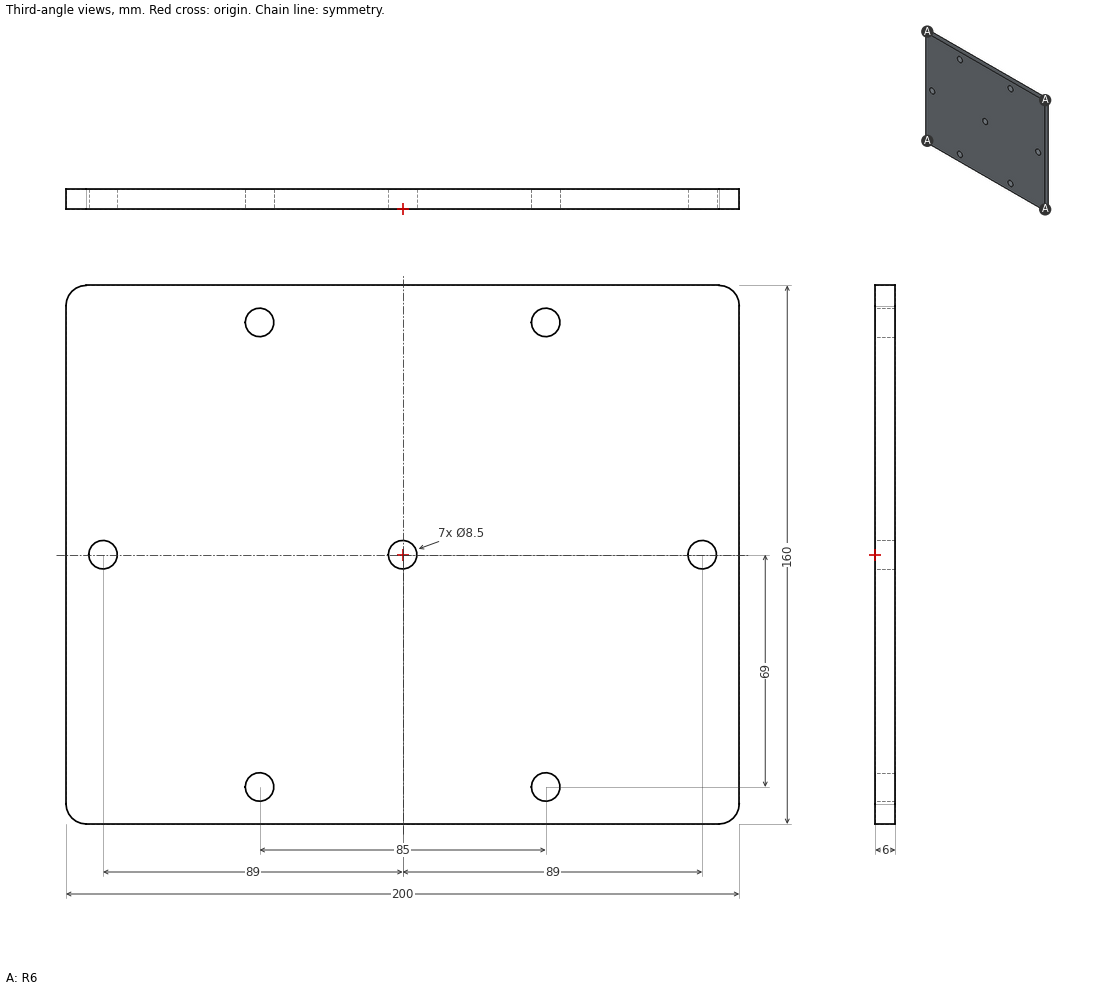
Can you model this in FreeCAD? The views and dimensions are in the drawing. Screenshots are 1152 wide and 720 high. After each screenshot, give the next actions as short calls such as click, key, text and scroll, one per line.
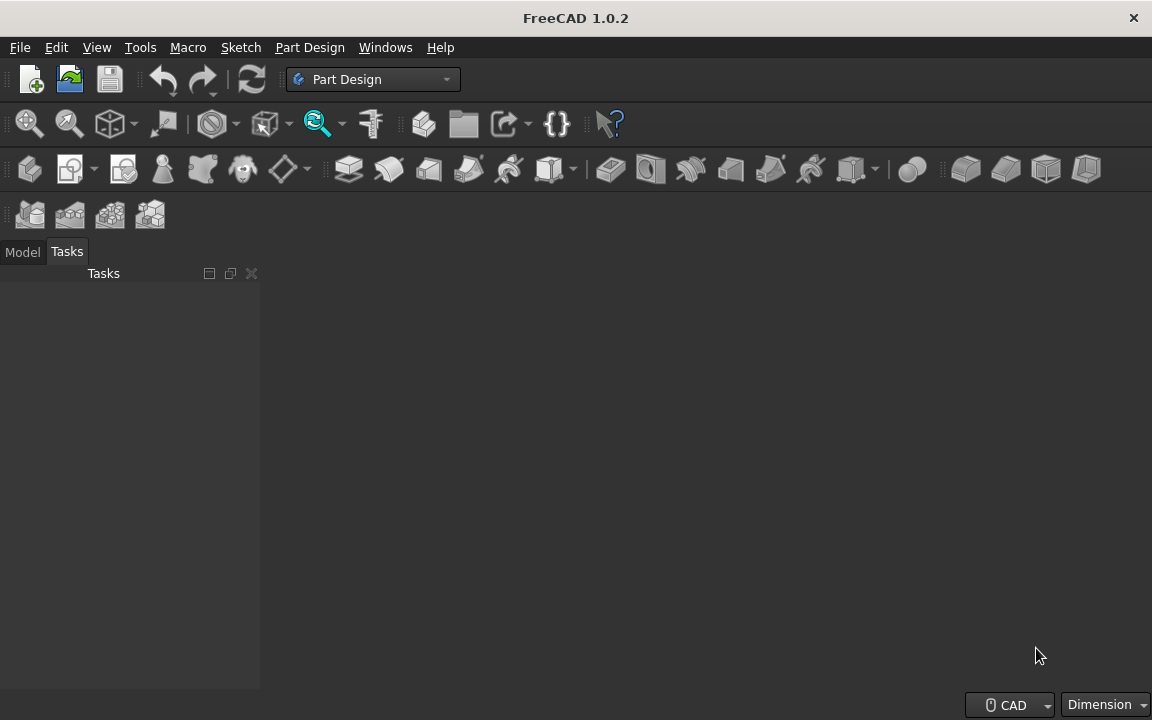
click(30, 80)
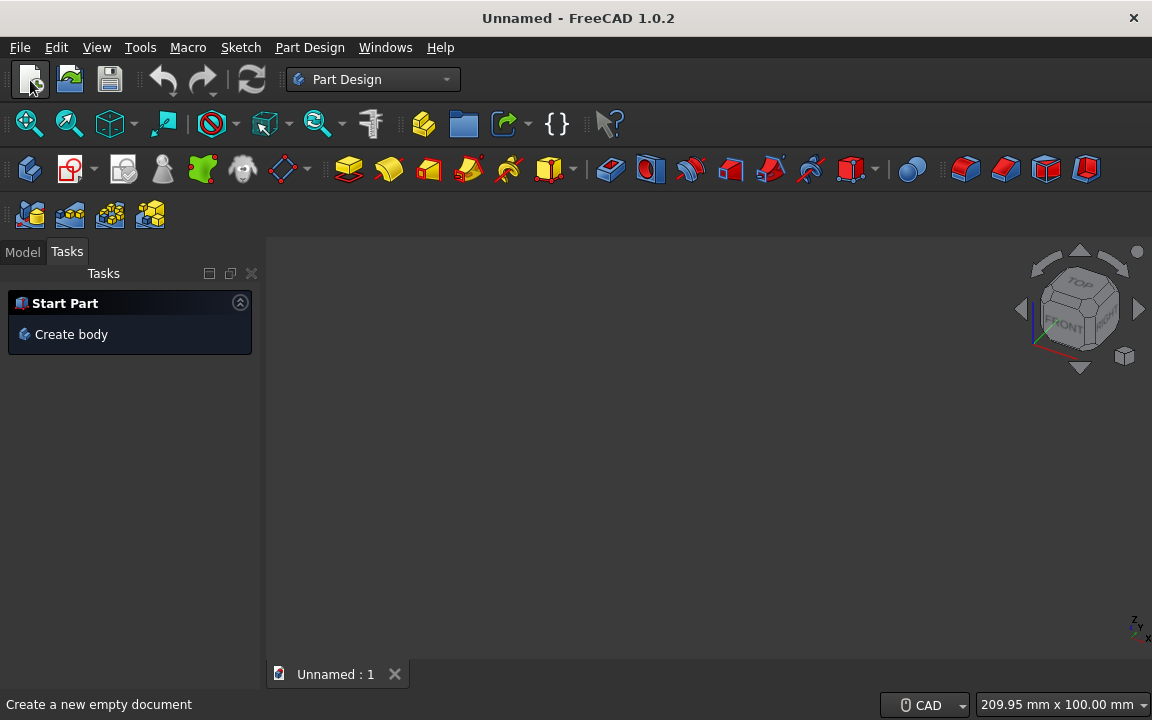
click(70, 170)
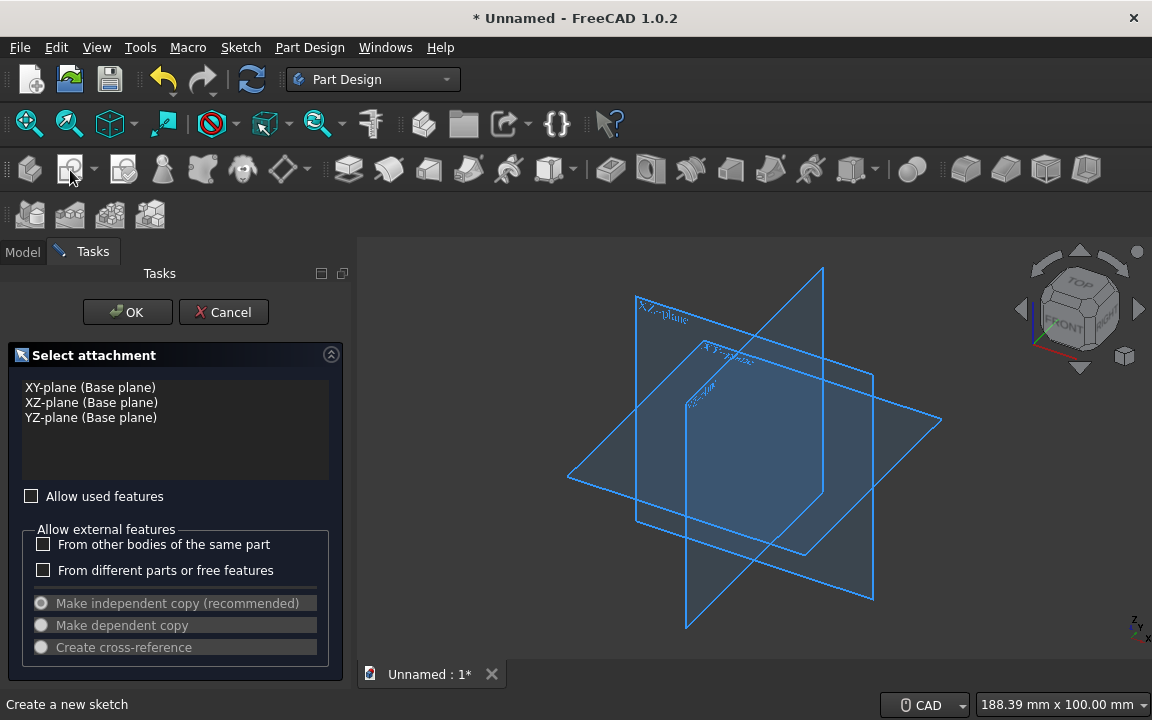
click(82, 402)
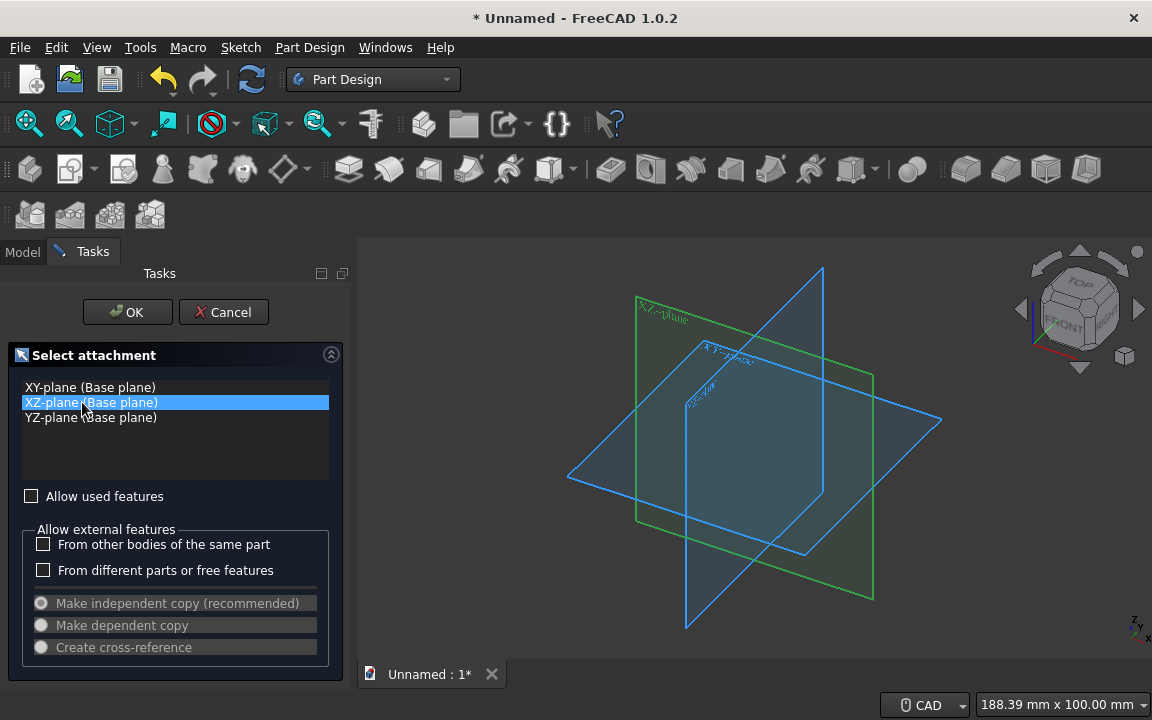
click(128, 312)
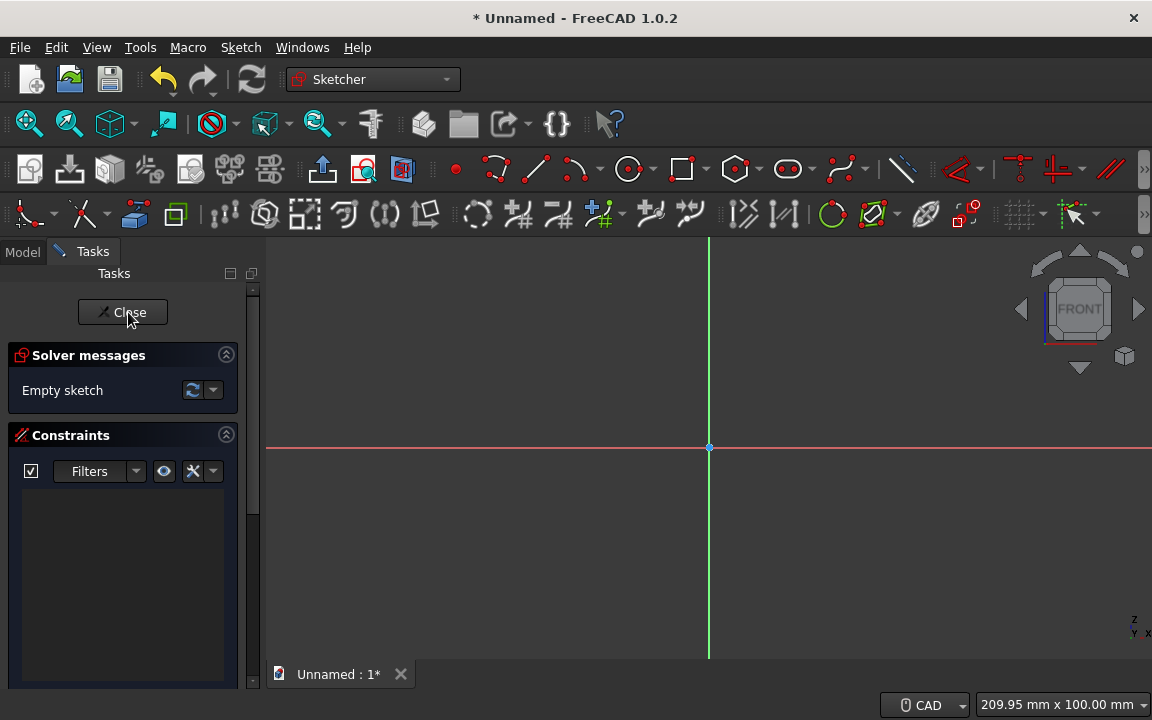
scroll(601, 448, down, 5)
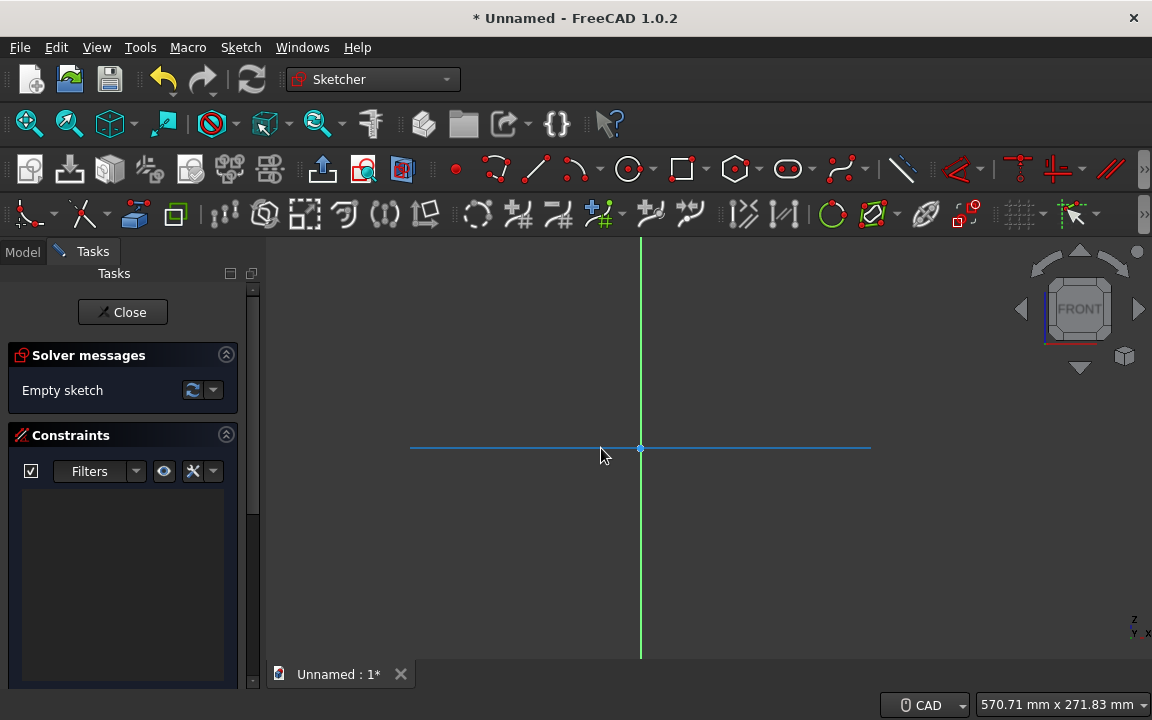
click(708, 170)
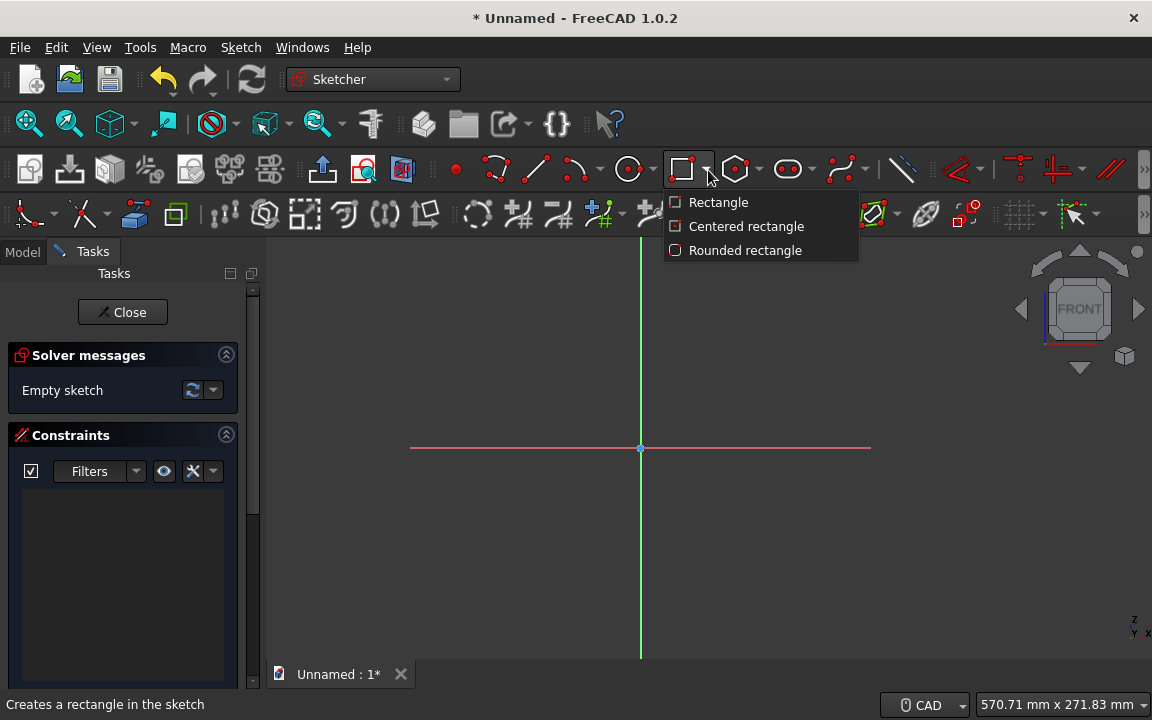
click(762, 226)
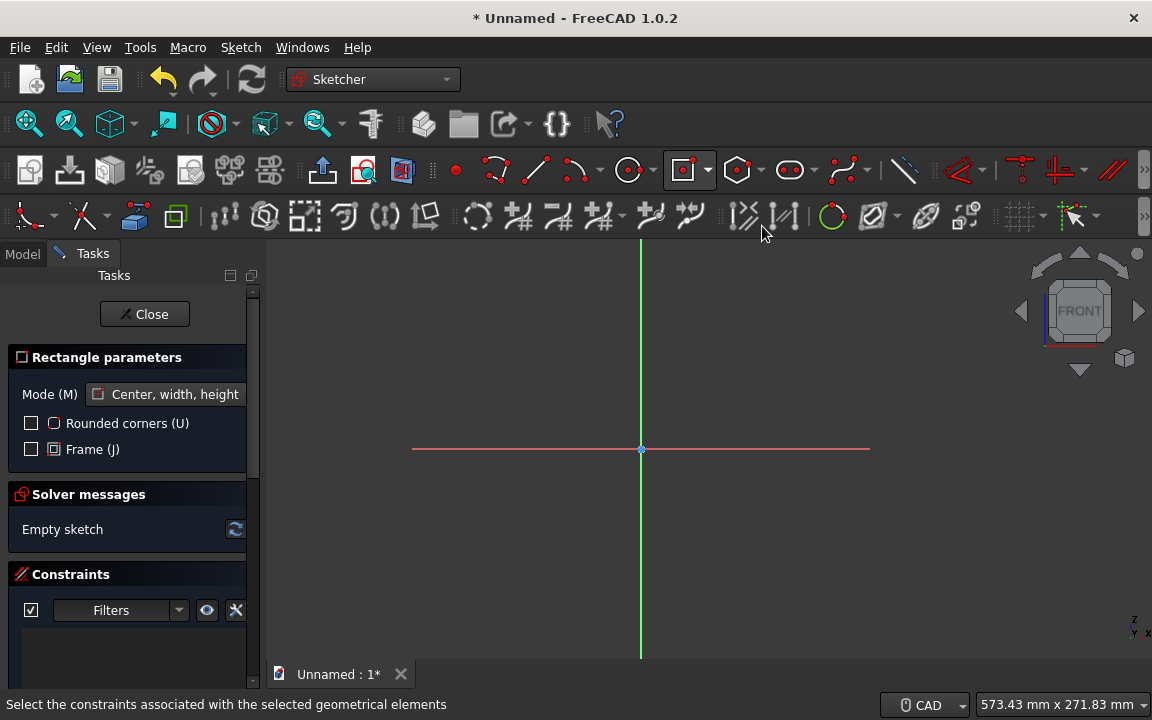
click(641, 449)
click(796, 326)
key(Escape)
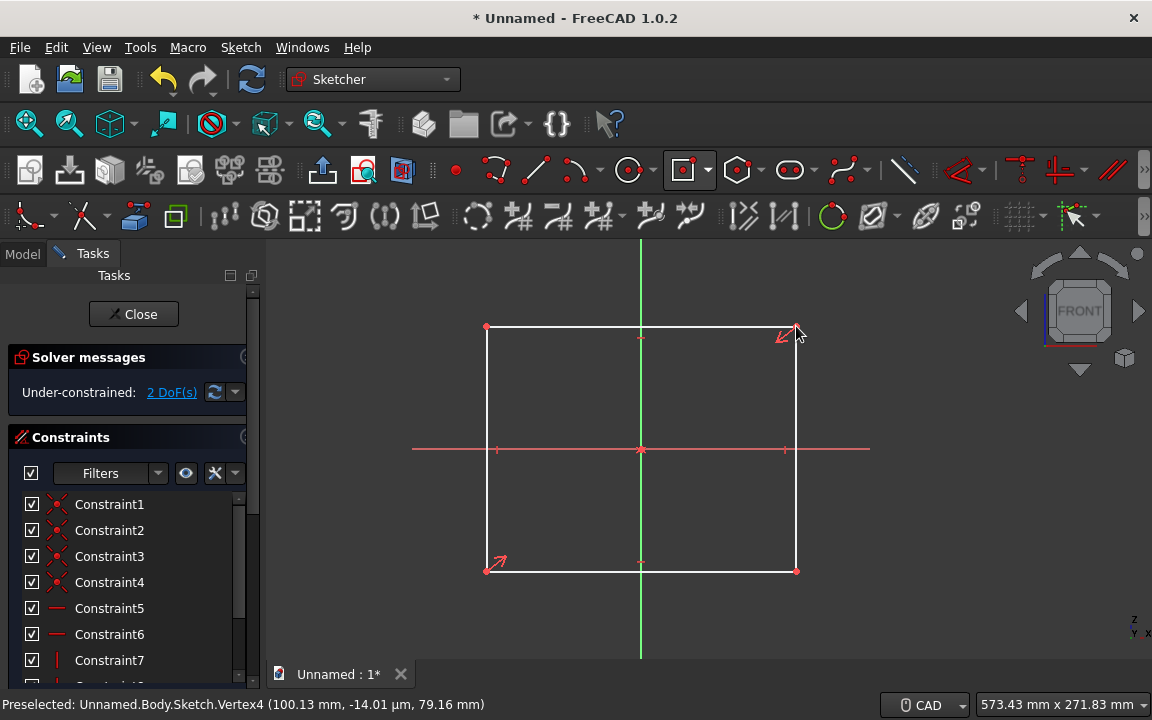
click(958, 170)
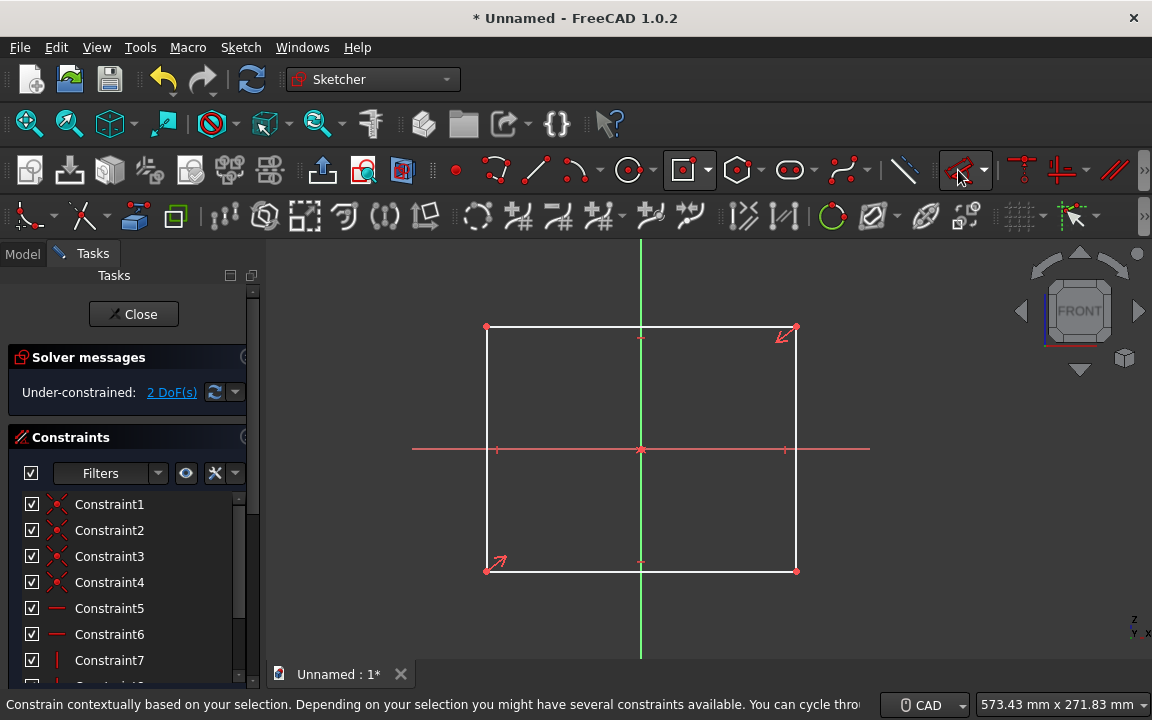
click(579, 572)
click(570, 606)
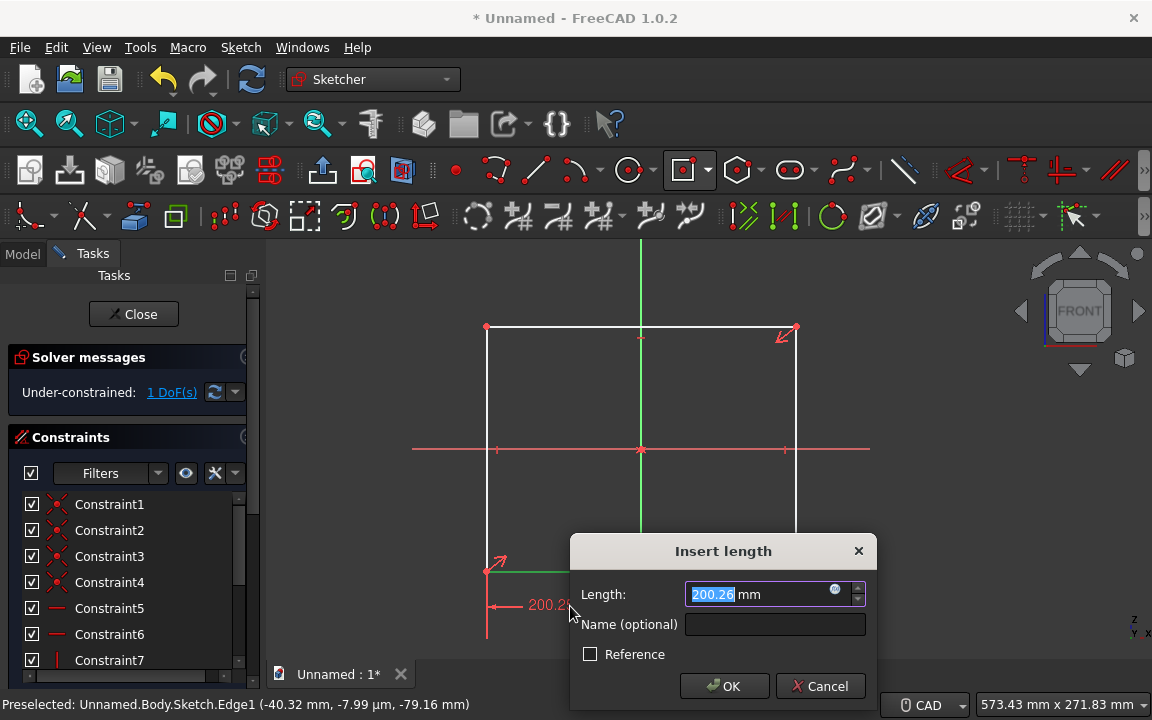
text(200)
key(Return)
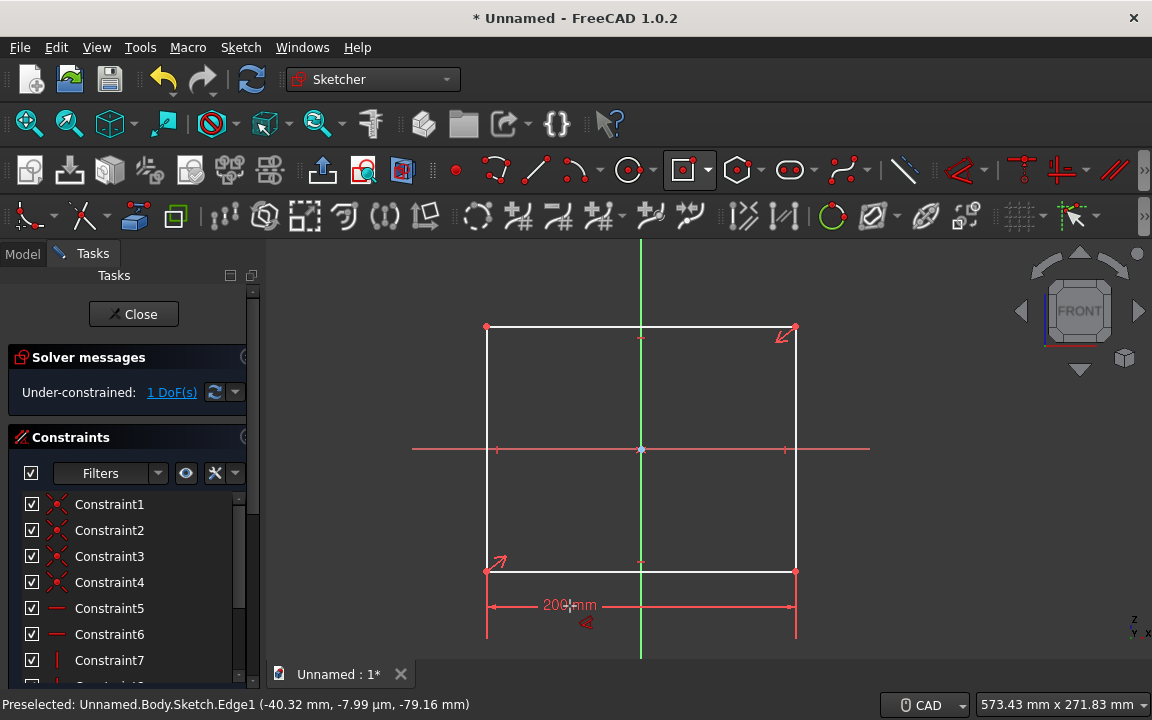
click(796, 498)
click(830, 393)